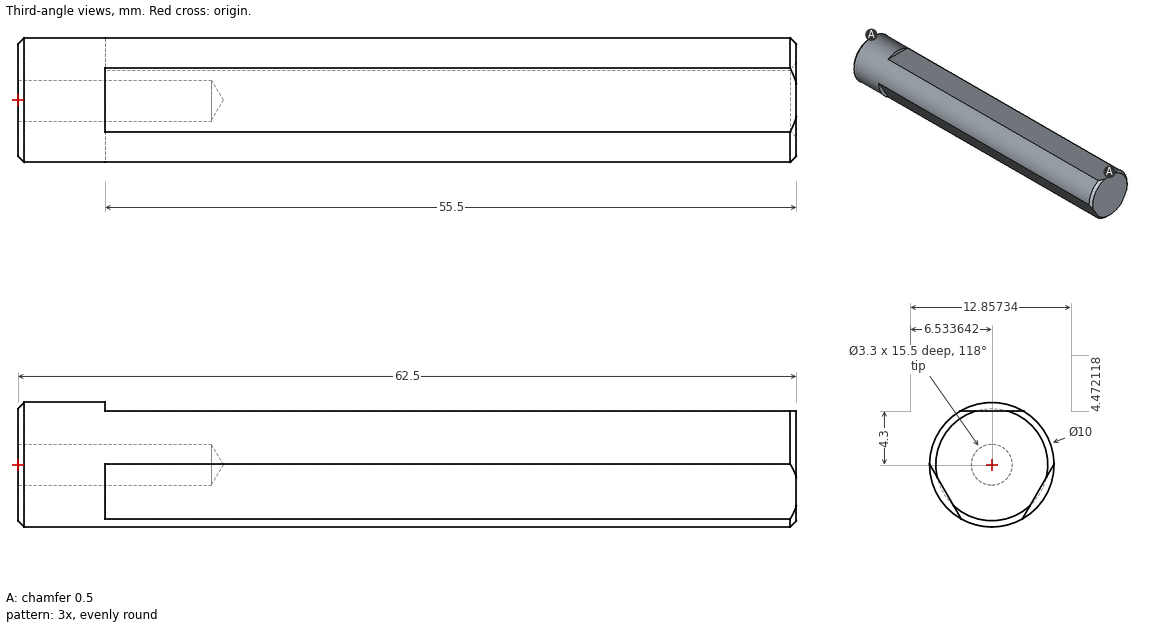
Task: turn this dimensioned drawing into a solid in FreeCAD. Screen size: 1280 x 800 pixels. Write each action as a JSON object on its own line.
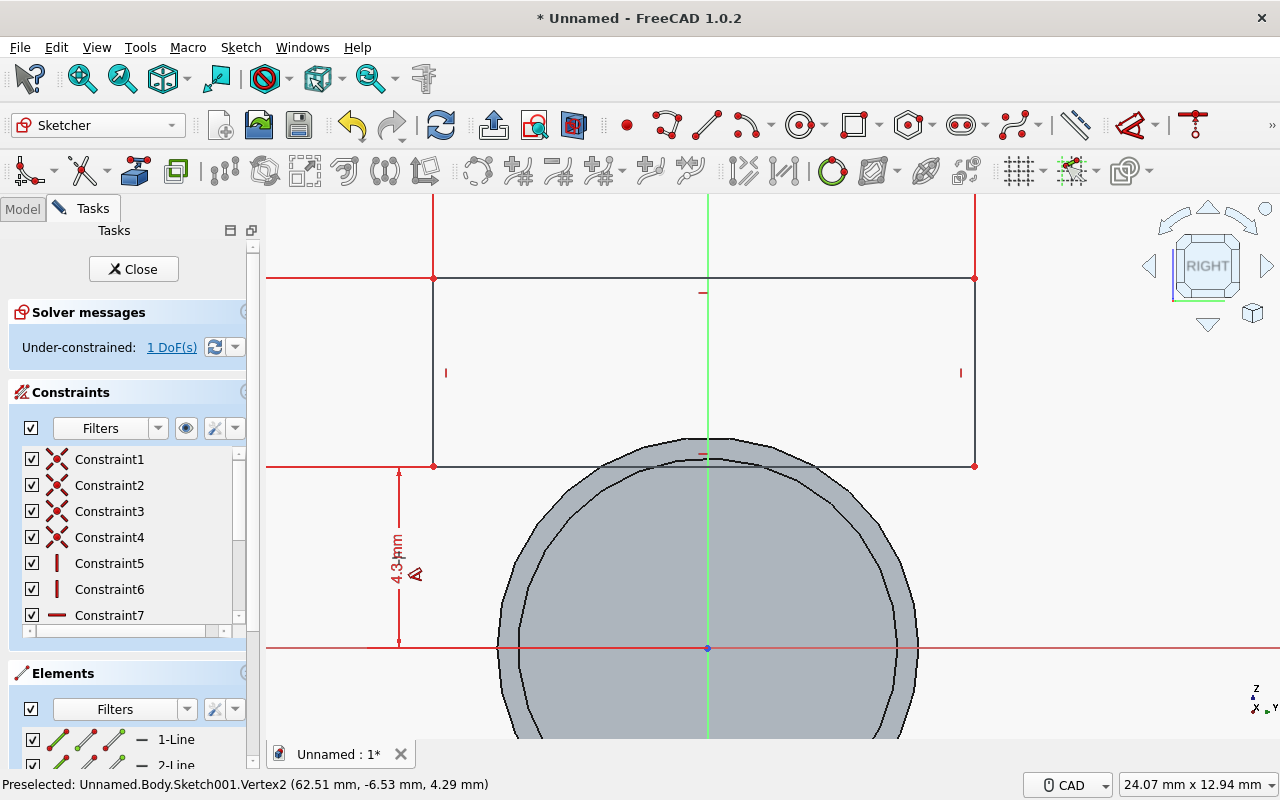
{"action": "left_click", "coordinate": [433, 278]}
{"action": "left_click", "coordinate": [570, 682]}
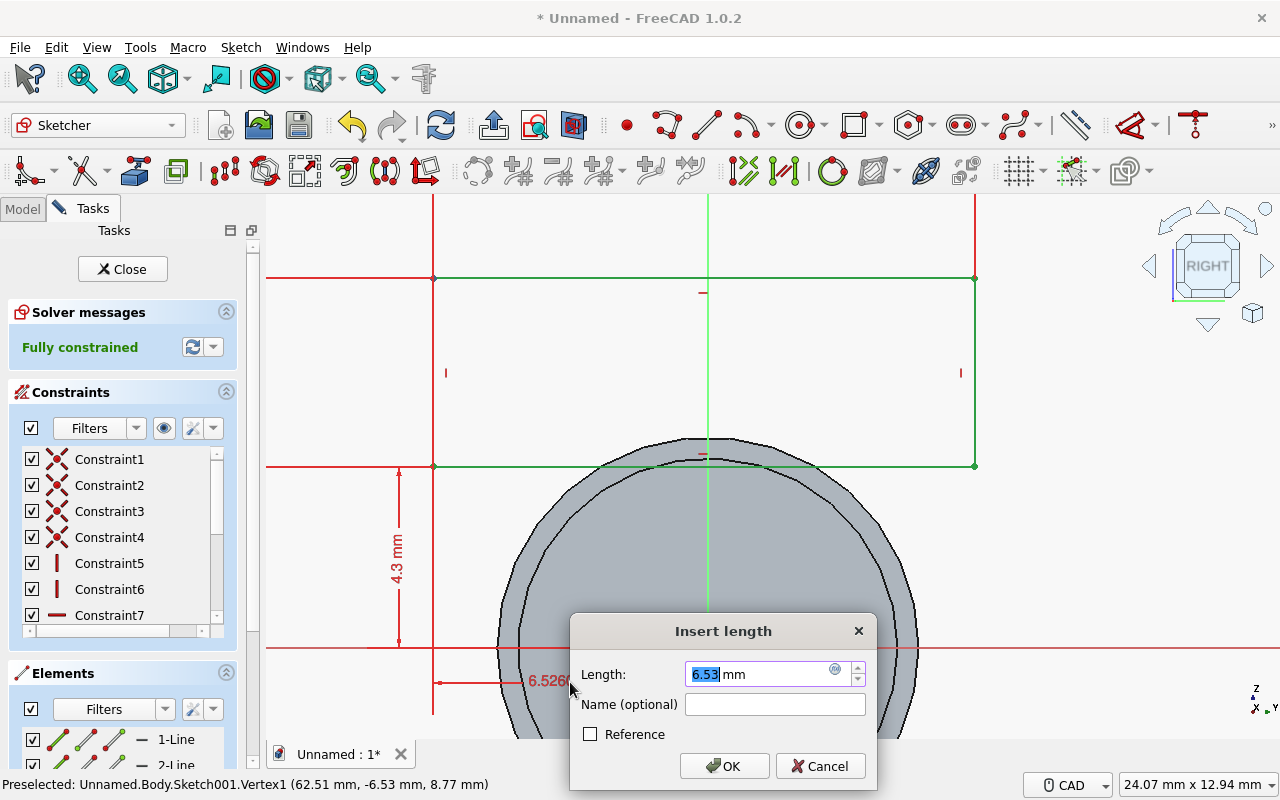
{"action": "type", "text": "6.533642"}
{"action": "key", "text": "Return"}
{"action": "key", "text": "Escape"}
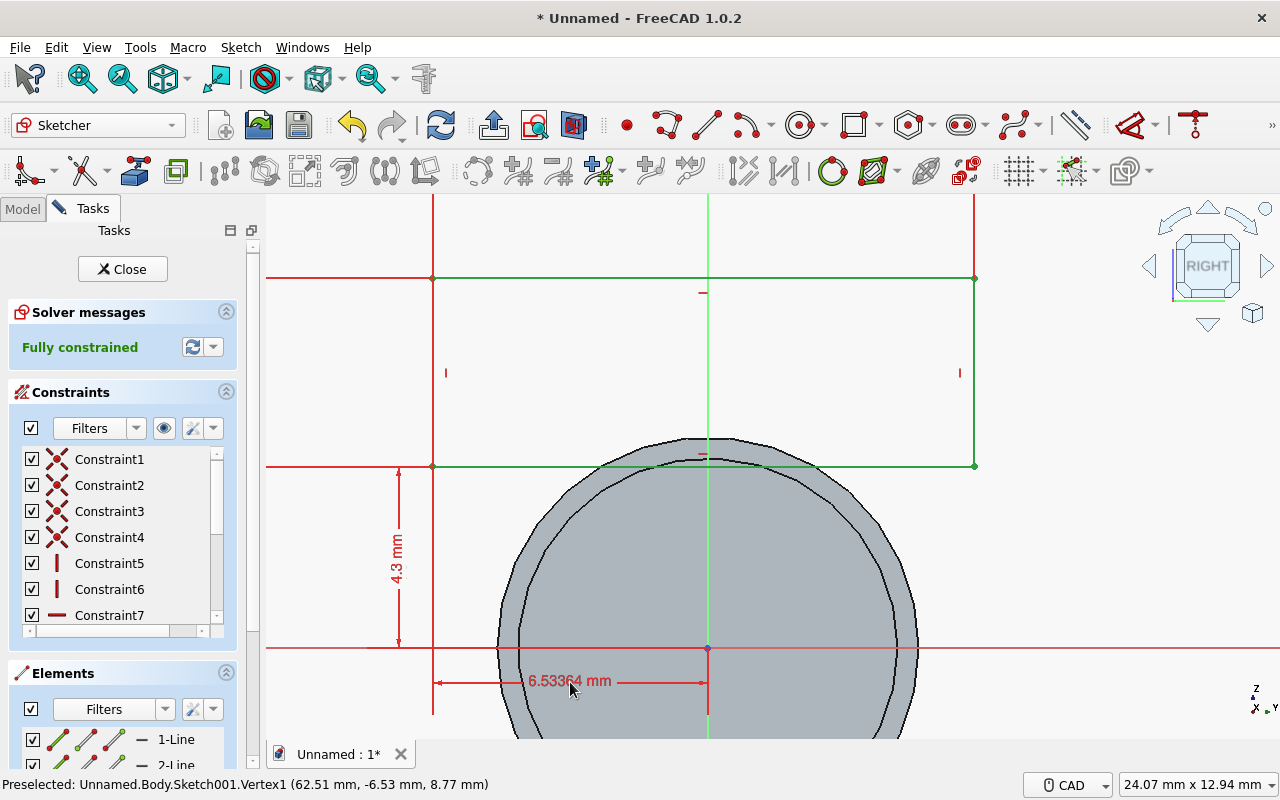
{"action": "left_click", "coordinate": [123, 269]}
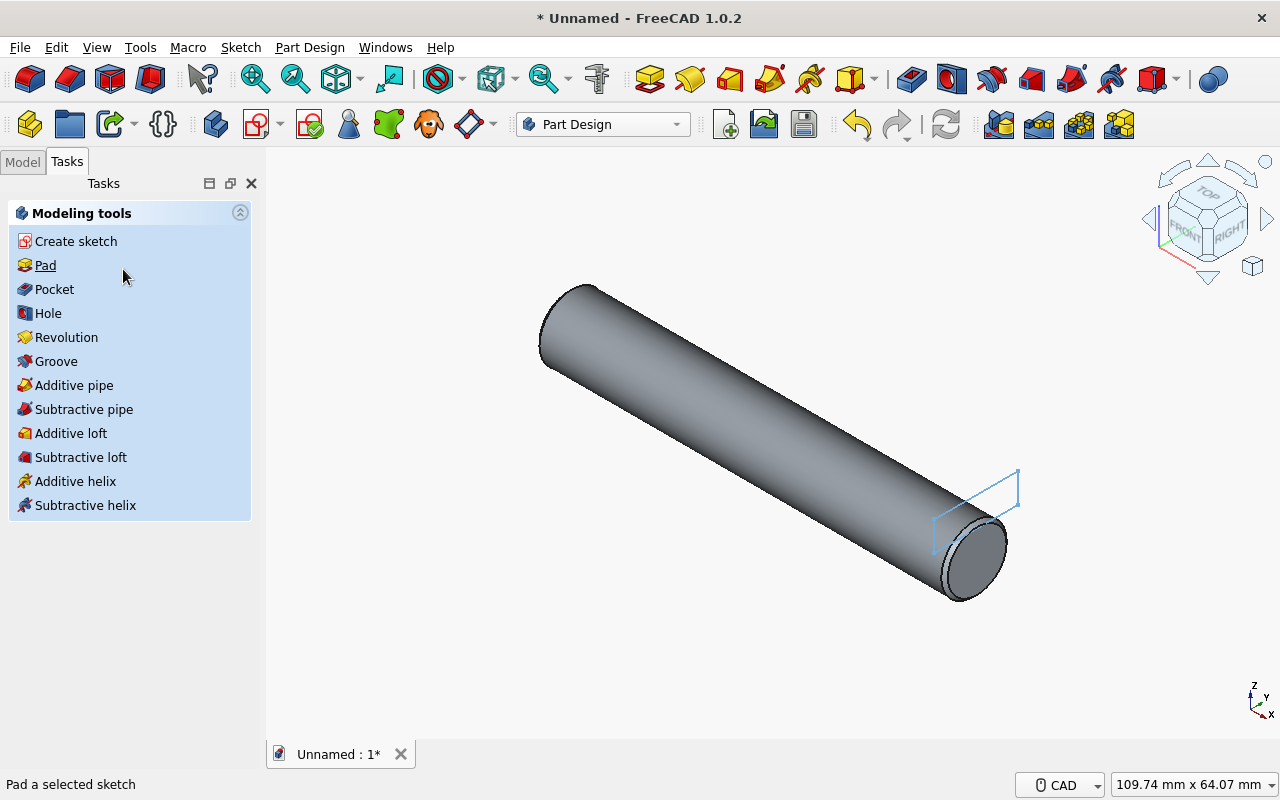
{"action": "left_click", "coordinate": [912, 80]}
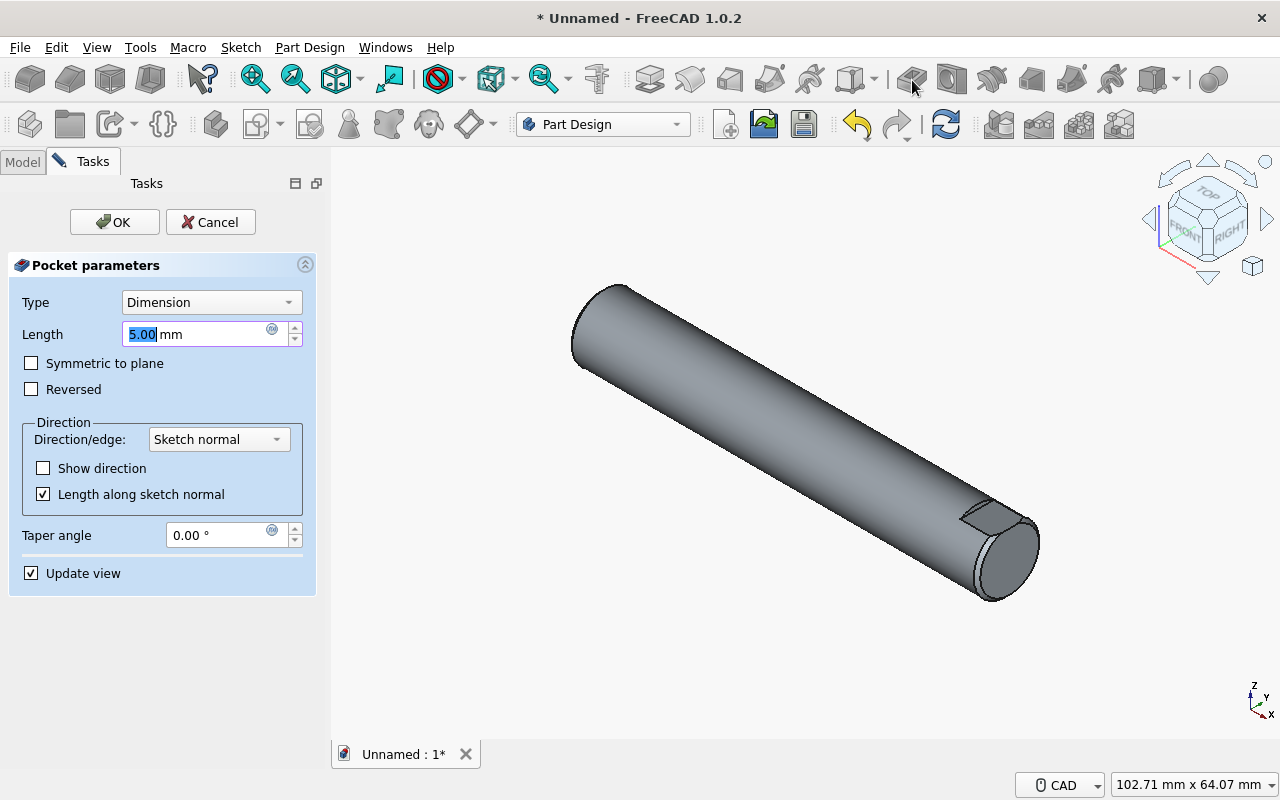
{"action": "type", "text": "55.5"}
{"action": "key", "text": "Tab"}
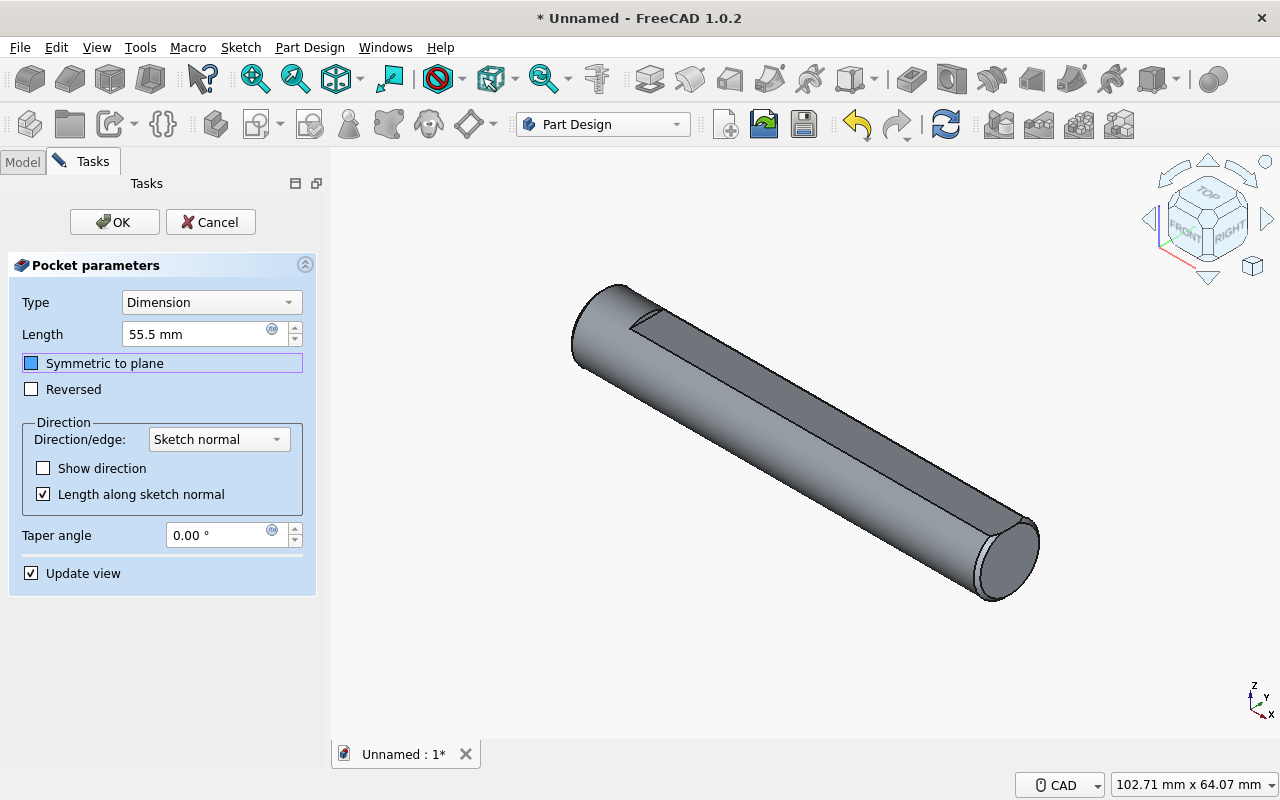
{"action": "left_click", "coordinate": [115, 222]}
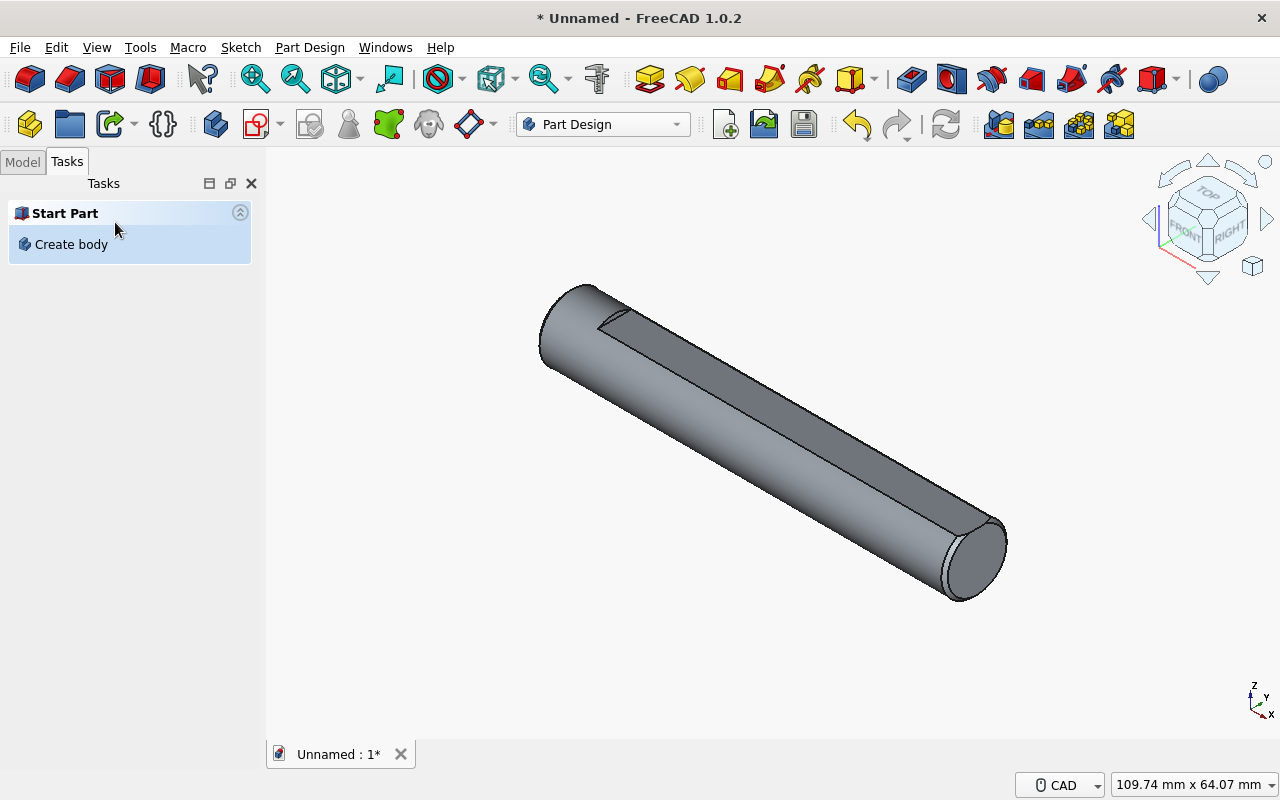
{"action": "left_click", "coordinate": [23, 161]}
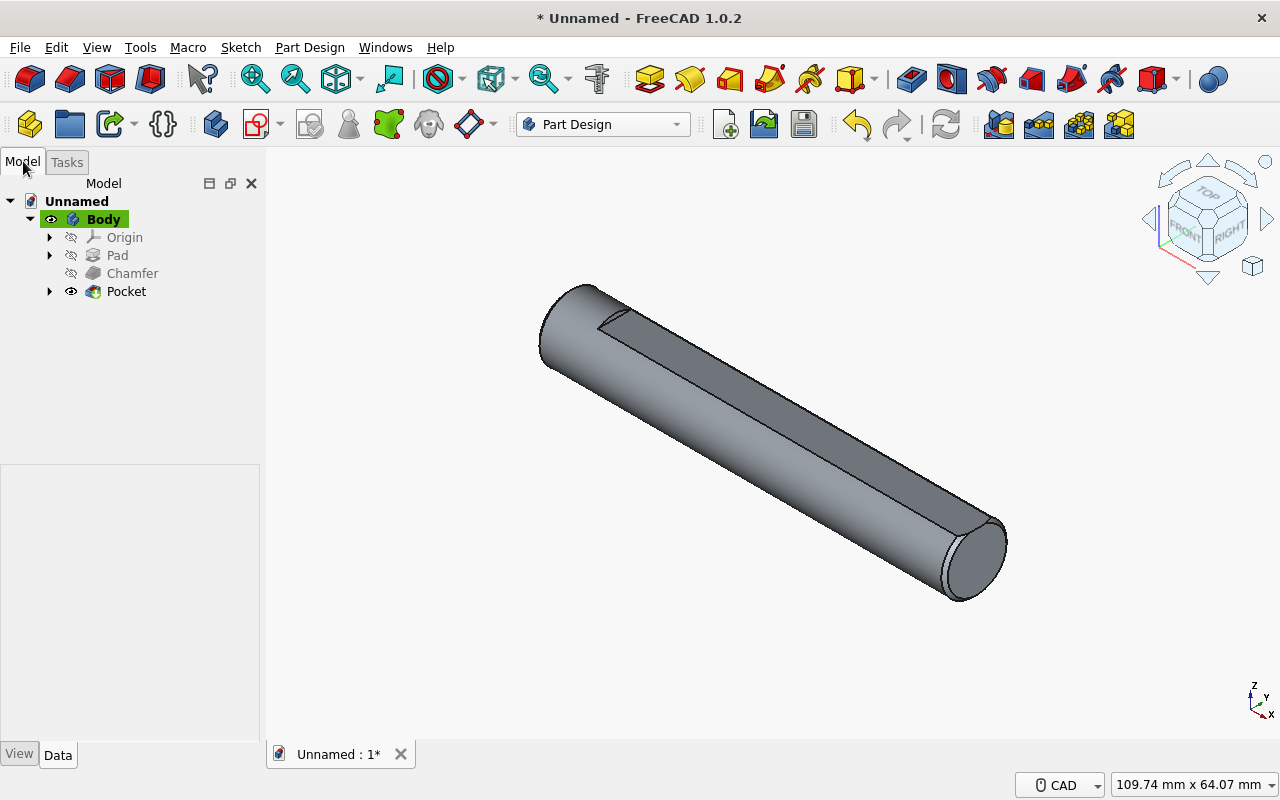
{"action": "left_click", "coordinate": [116, 291]}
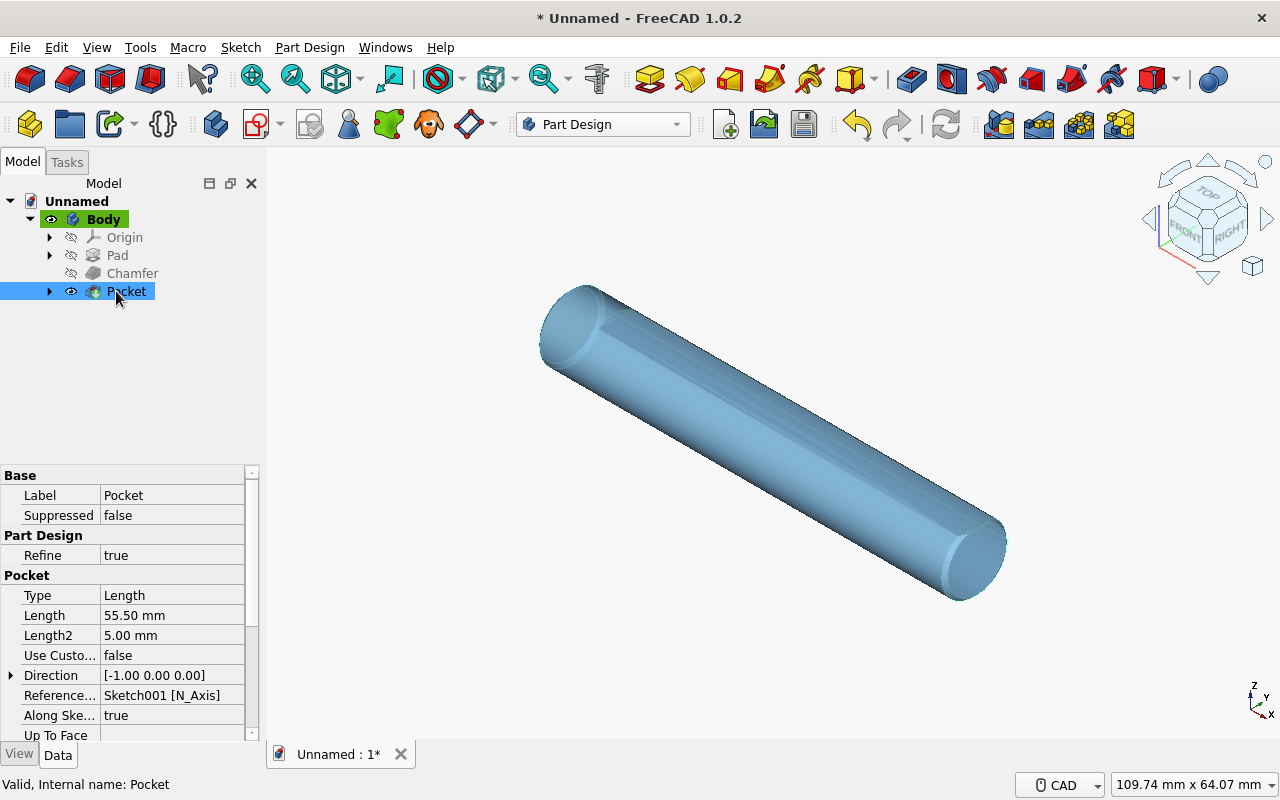
{"action": "left_click", "coordinate": [1080, 124]}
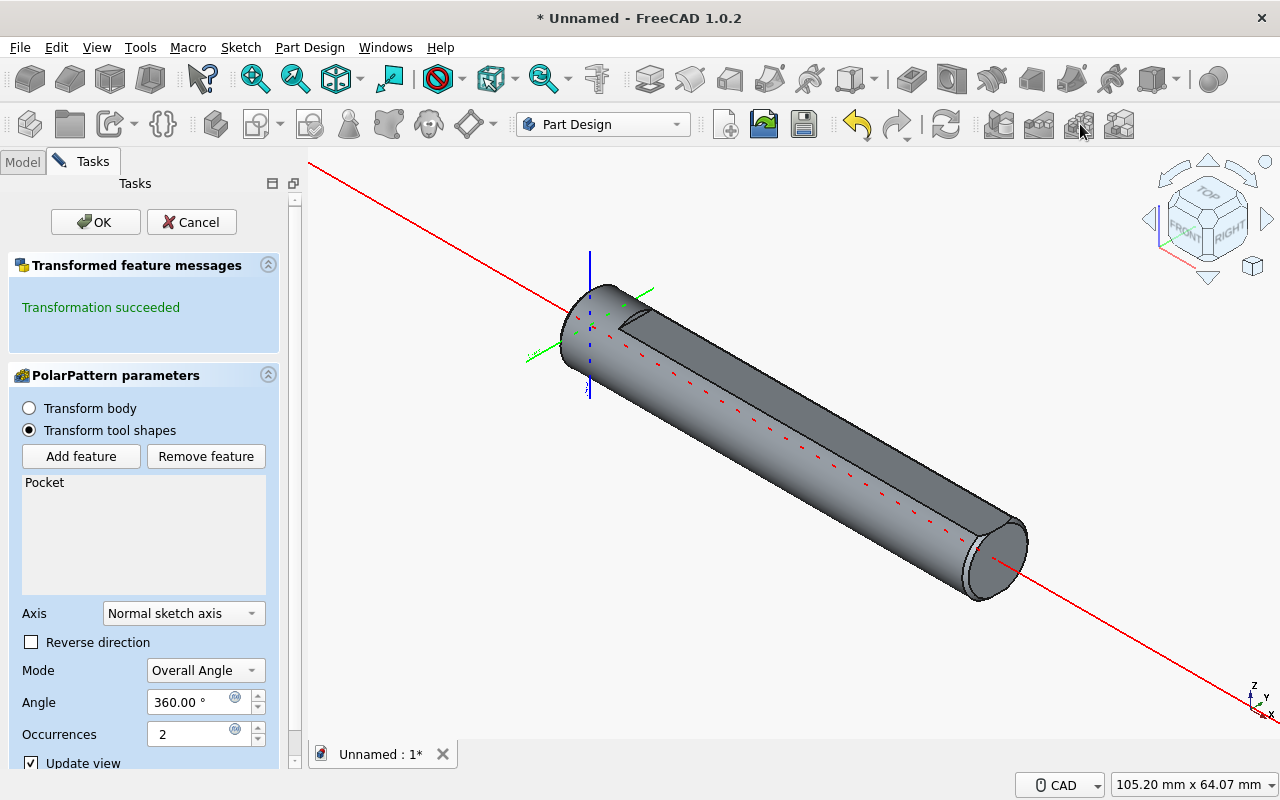
{"action": "left_click", "coordinate": [184, 614]}